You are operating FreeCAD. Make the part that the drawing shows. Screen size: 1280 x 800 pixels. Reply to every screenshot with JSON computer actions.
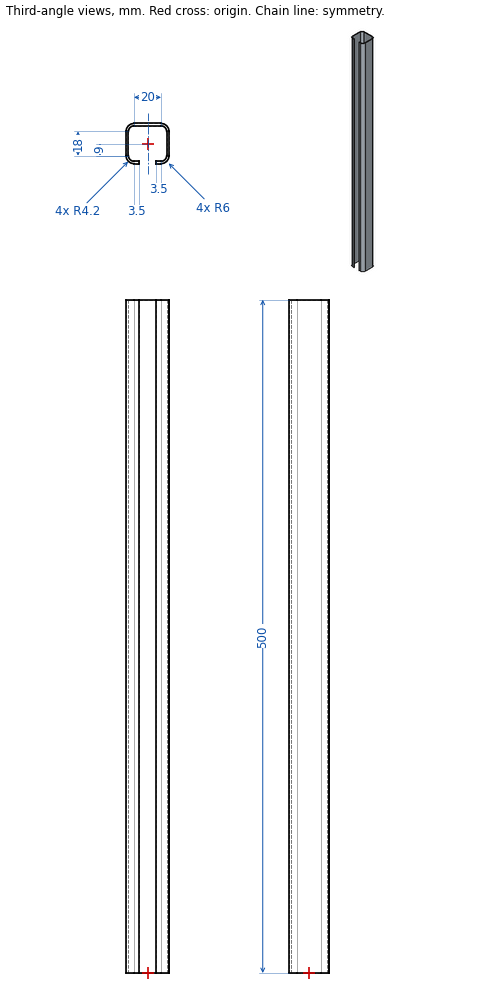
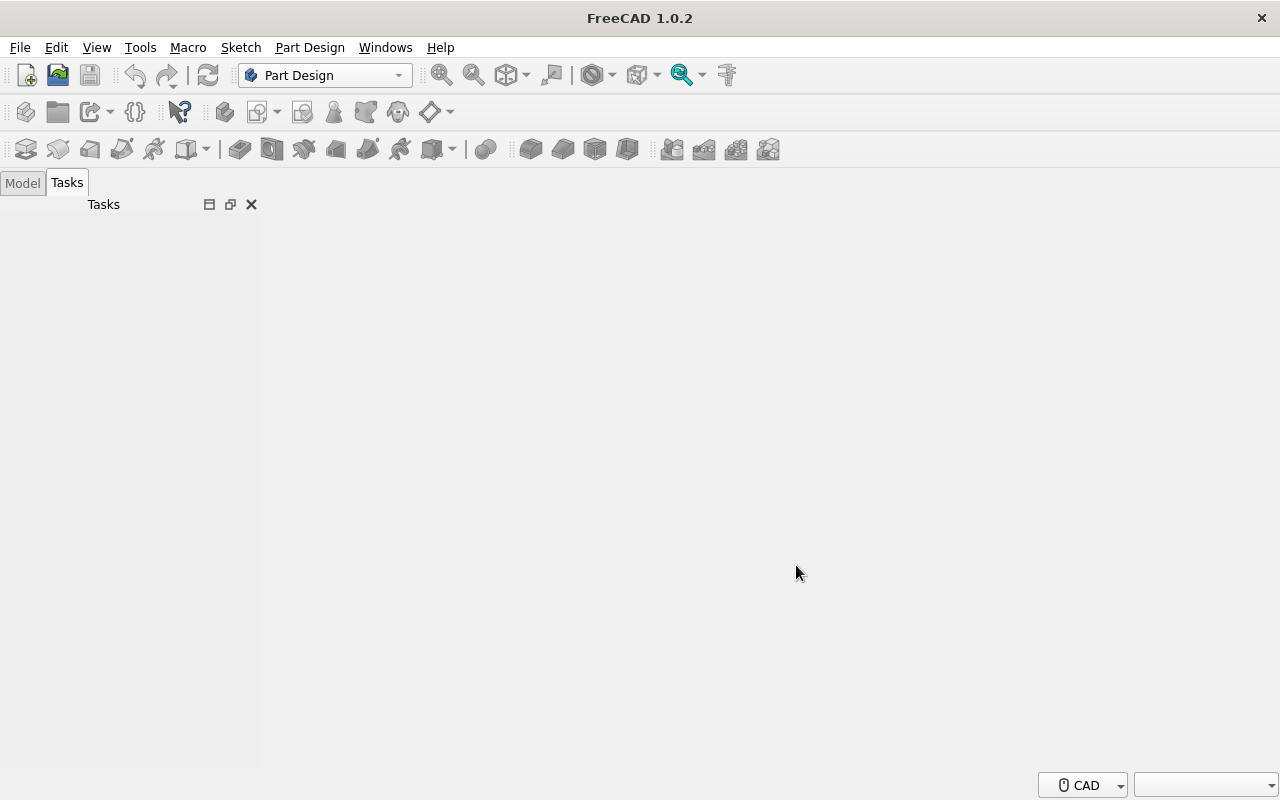
{"action": "left_click", "coordinate": [26, 76]}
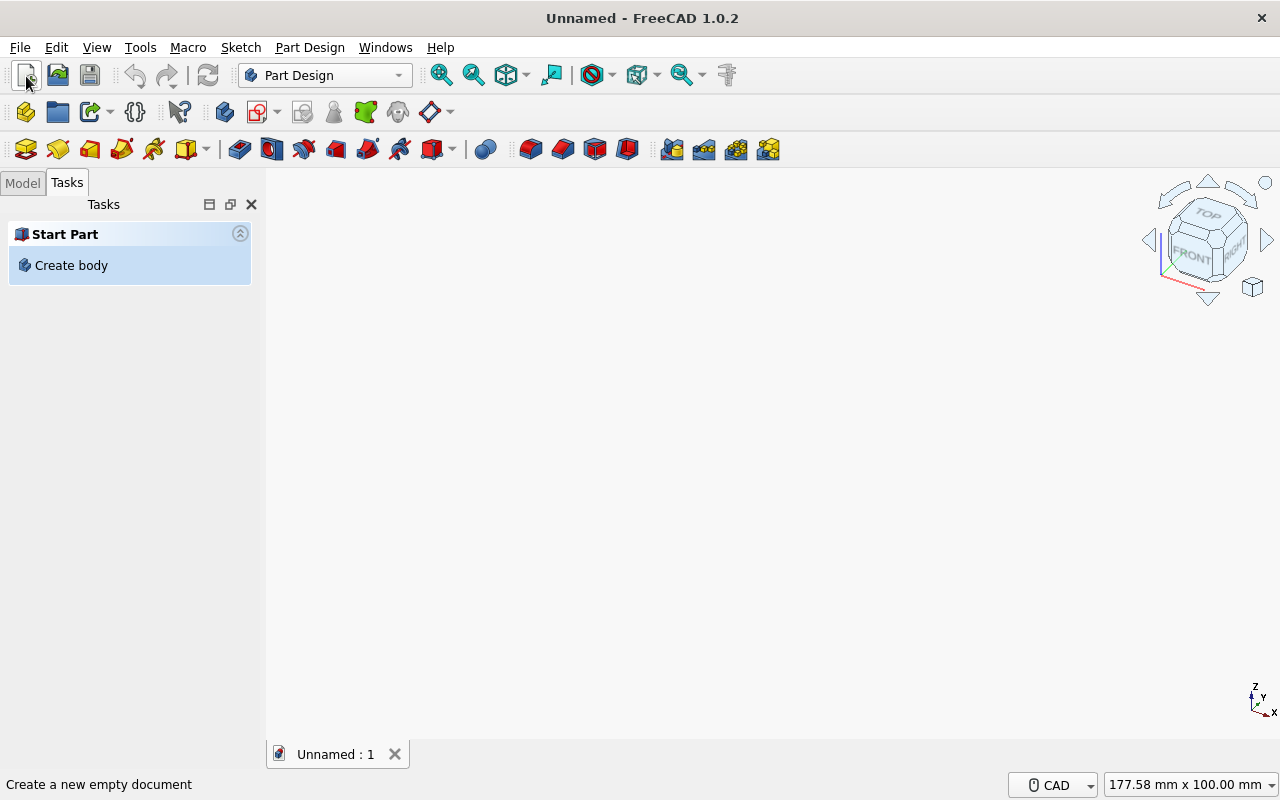
{"action": "left_click", "coordinate": [258, 112]}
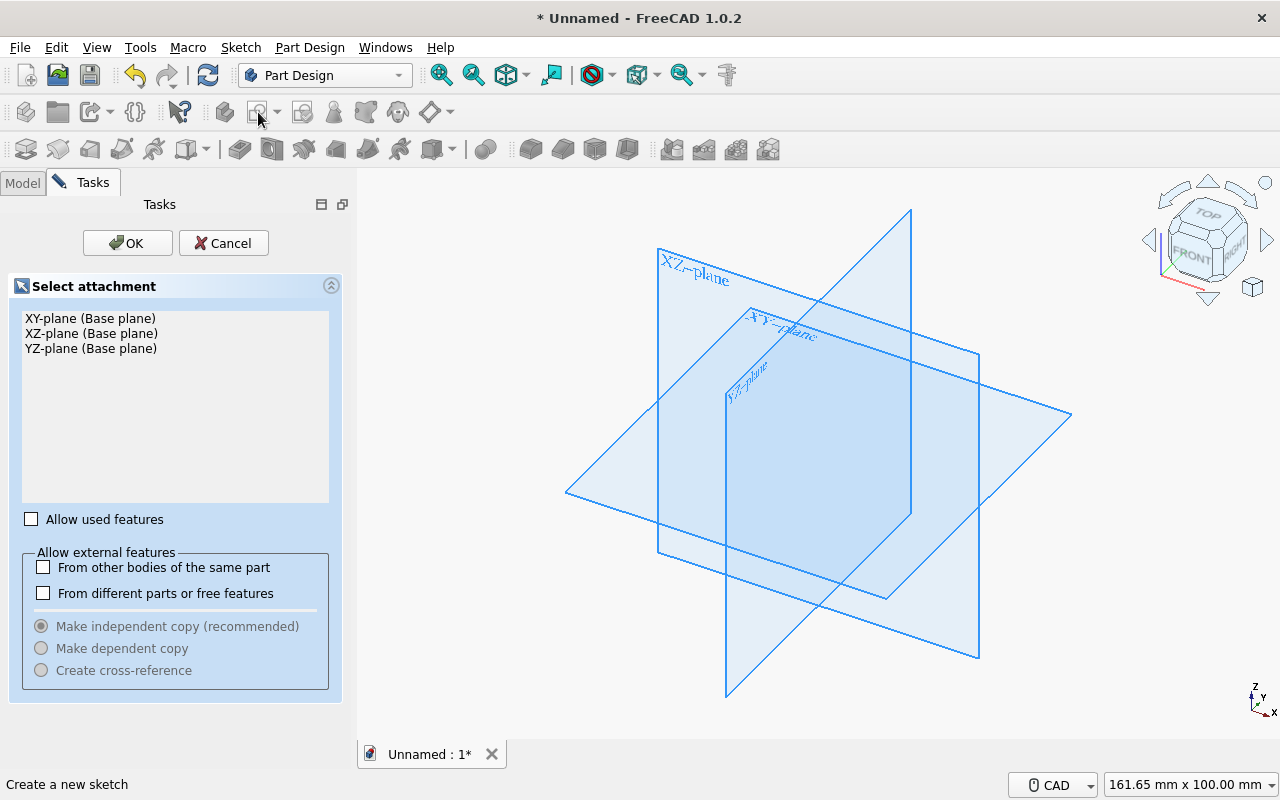
{"action": "left_click", "coordinate": [82, 318]}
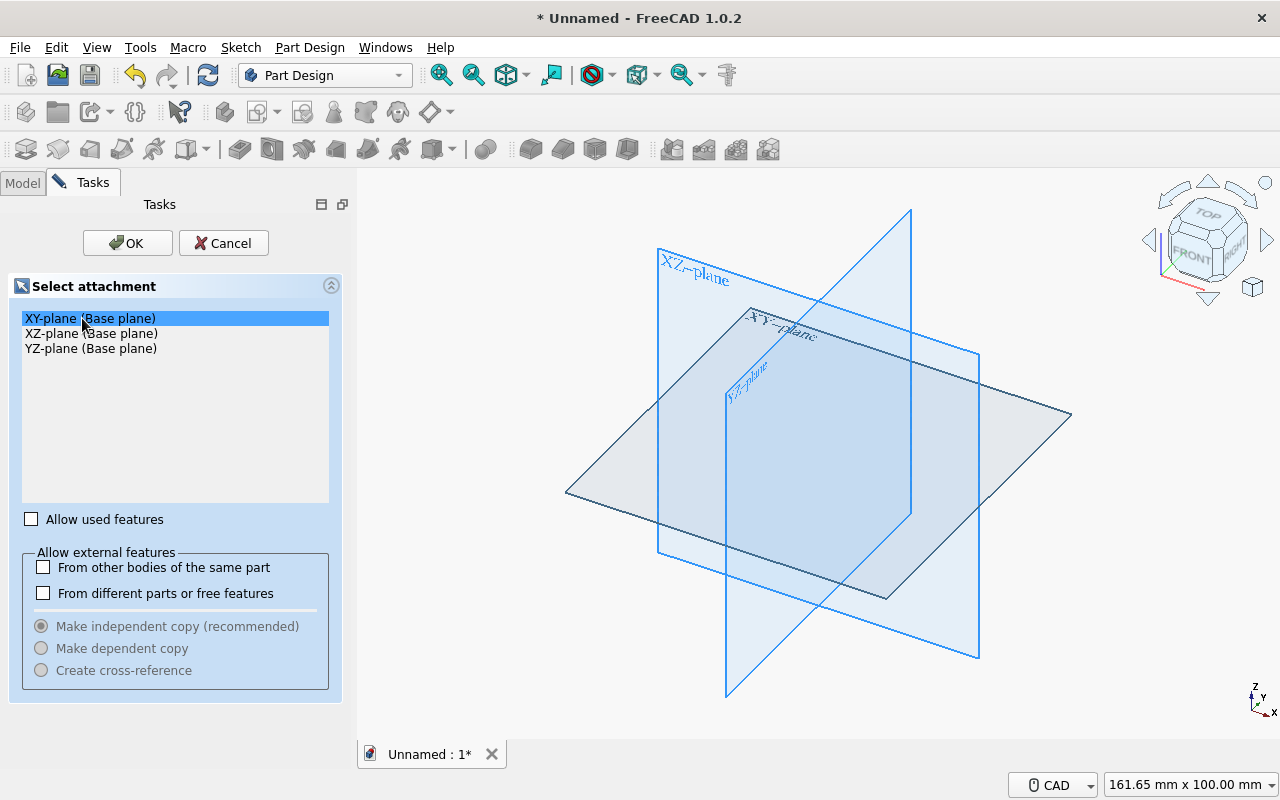
{"action": "left_click", "coordinate": [128, 243]}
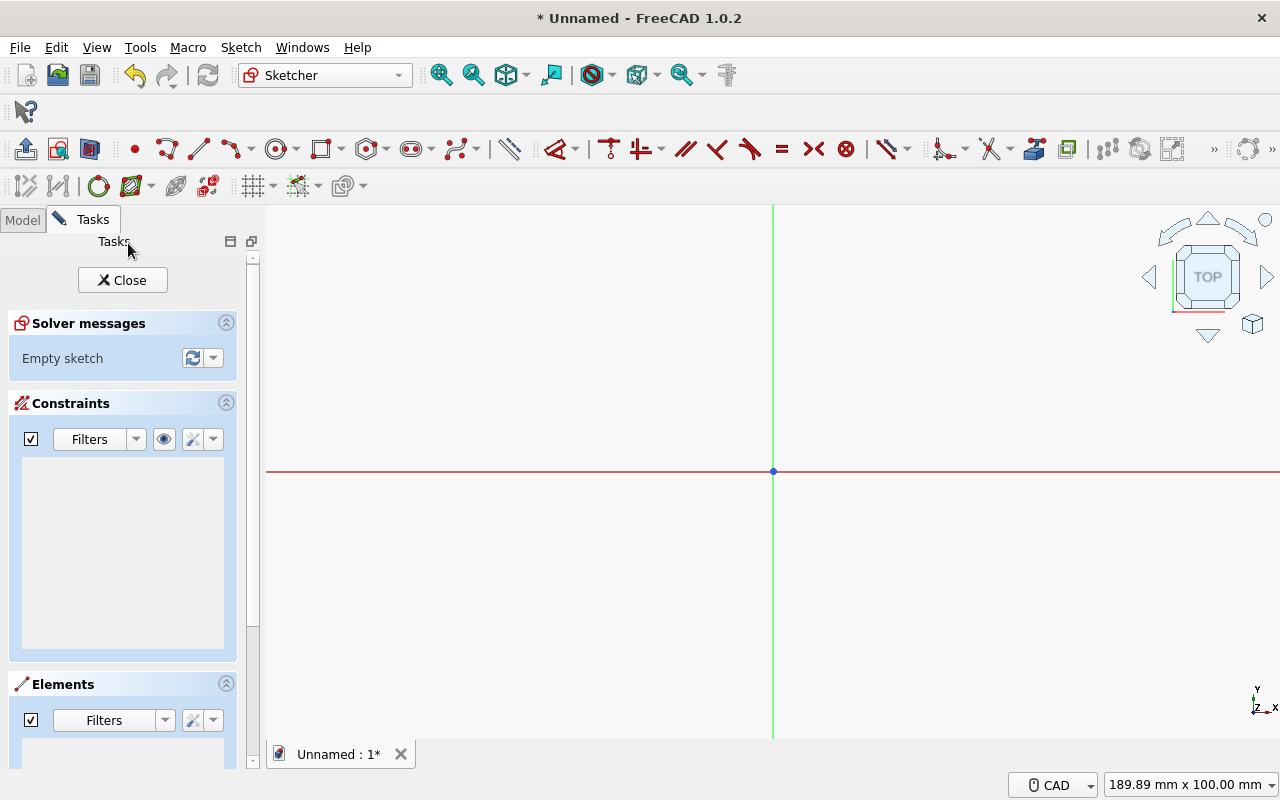
{"action": "scroll", "coordinate": [829, 472], "scroll_direction": "up", "scroll_amount": 4}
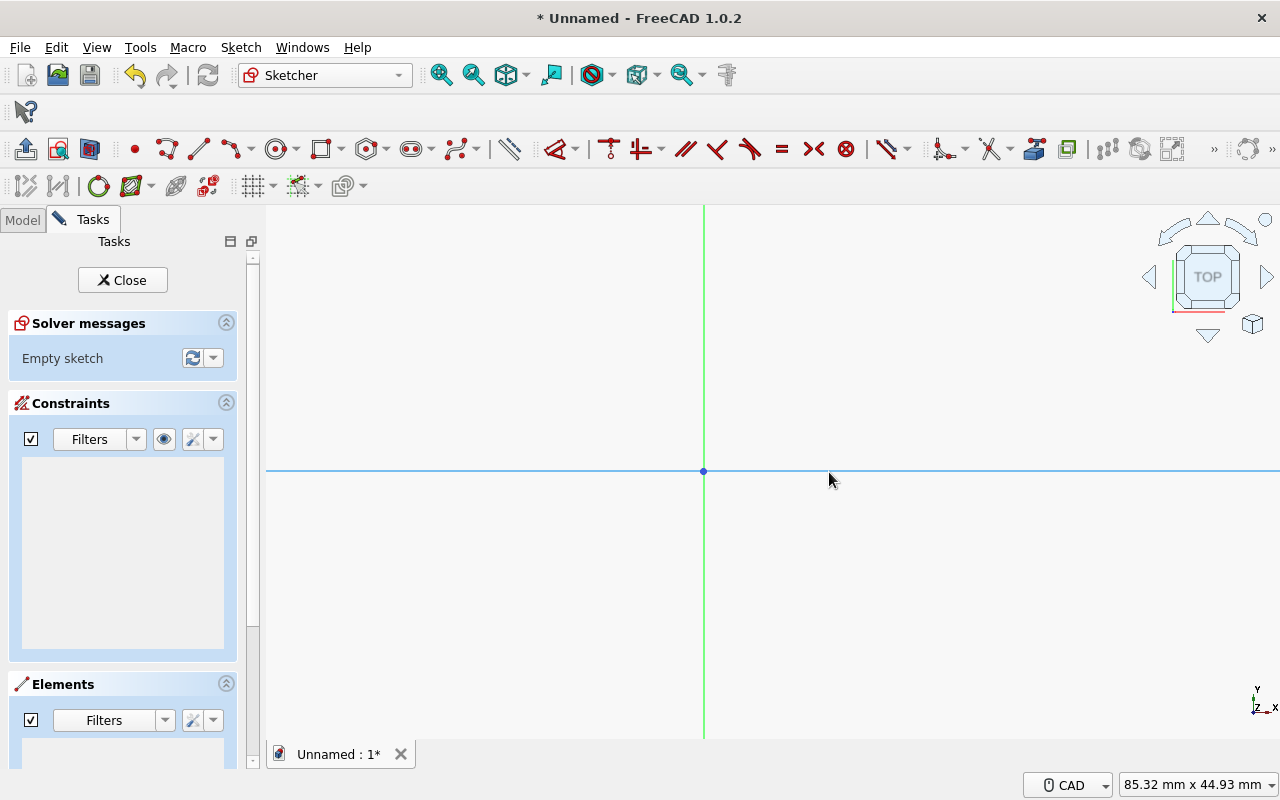
{"action": "left_click", "coordinate": [200, 150]}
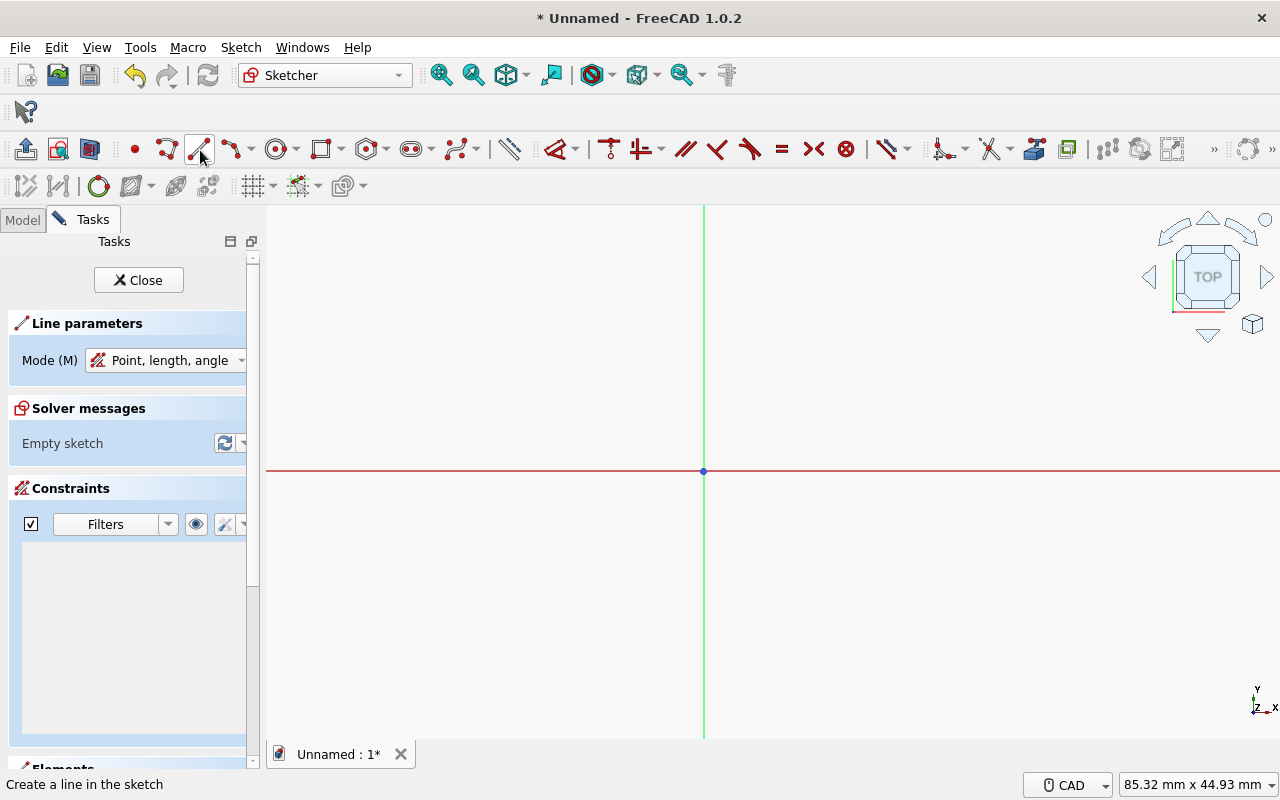
{"action": "left_click", "coordinate": [535, 578]}
{"action": "left_click", "coordinate": [535, 364]}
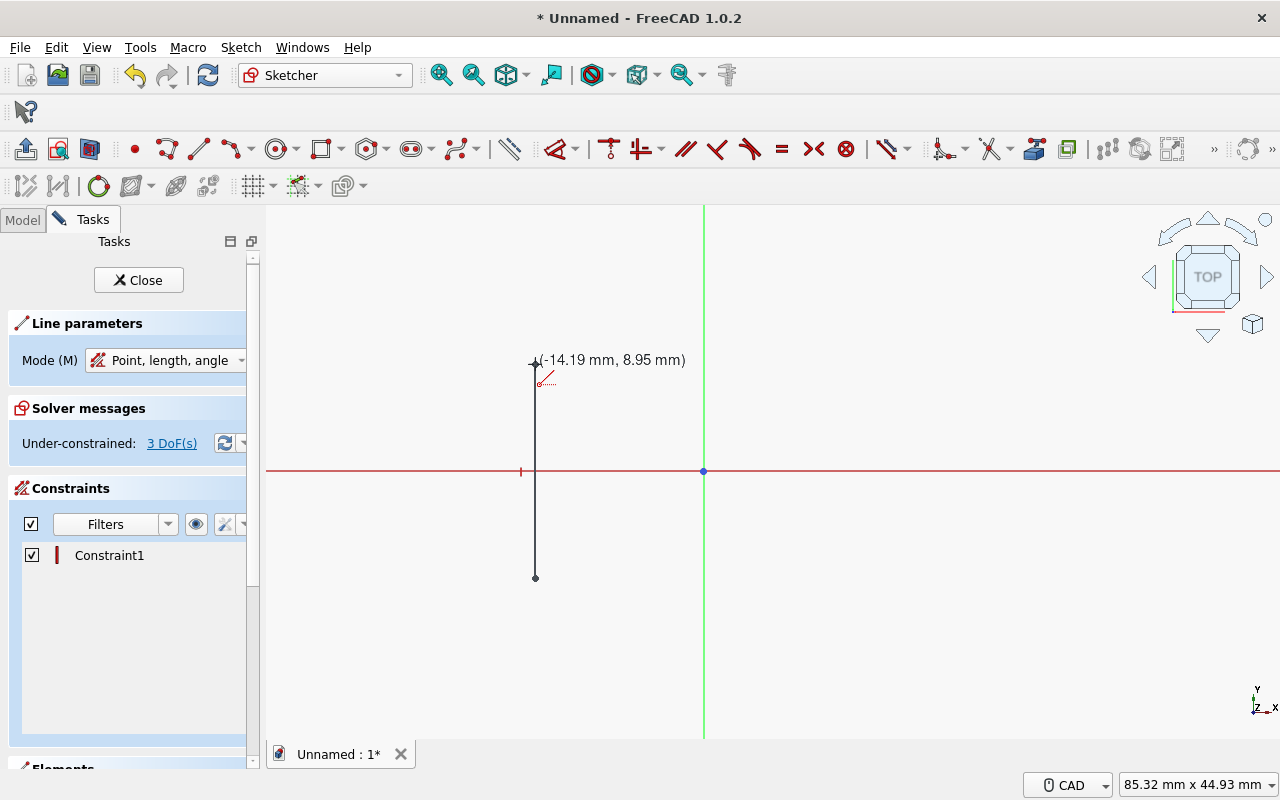
{"action": "left_click", "coordinate": [585, 315]}
{"action": "left_click", "coordinate": [823, 315]}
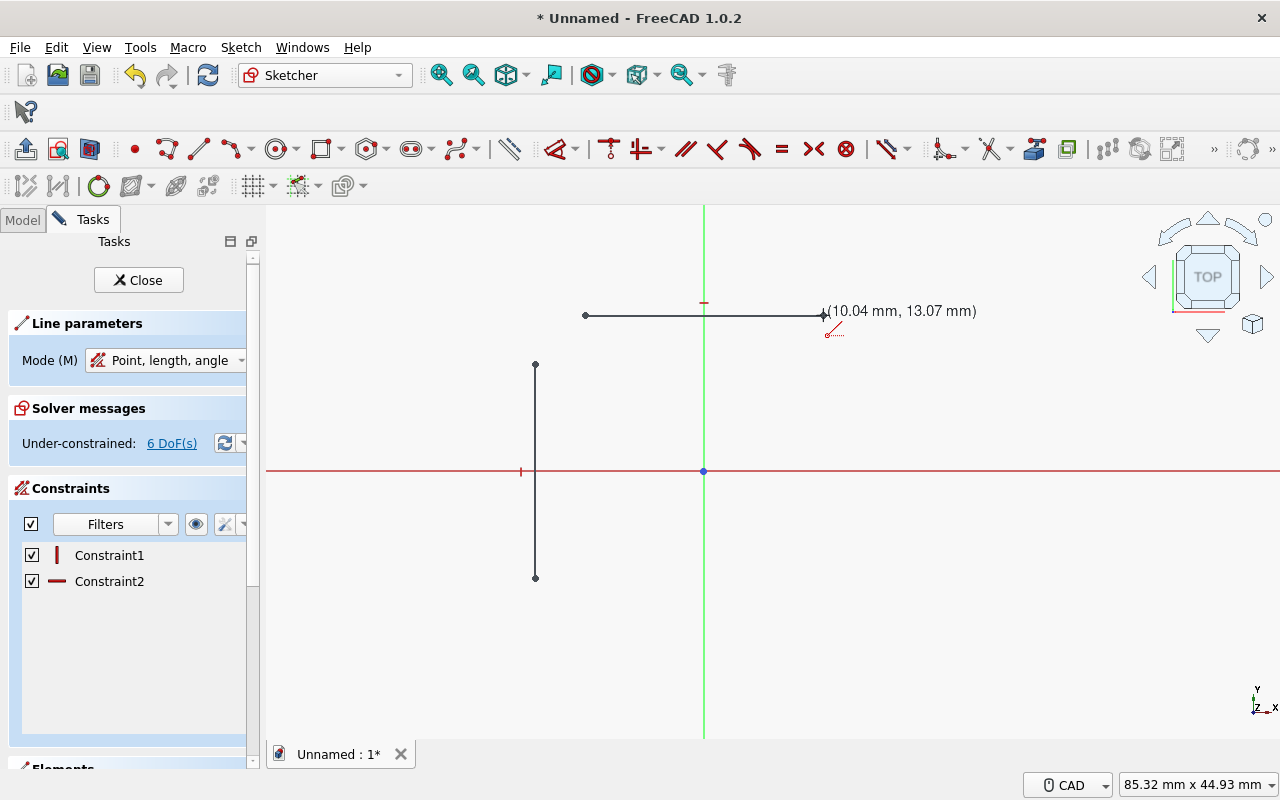
{"action": "left_click", "coordinate": [872, 364]}
{"action": "left_click", "coordinate": [872, 578]}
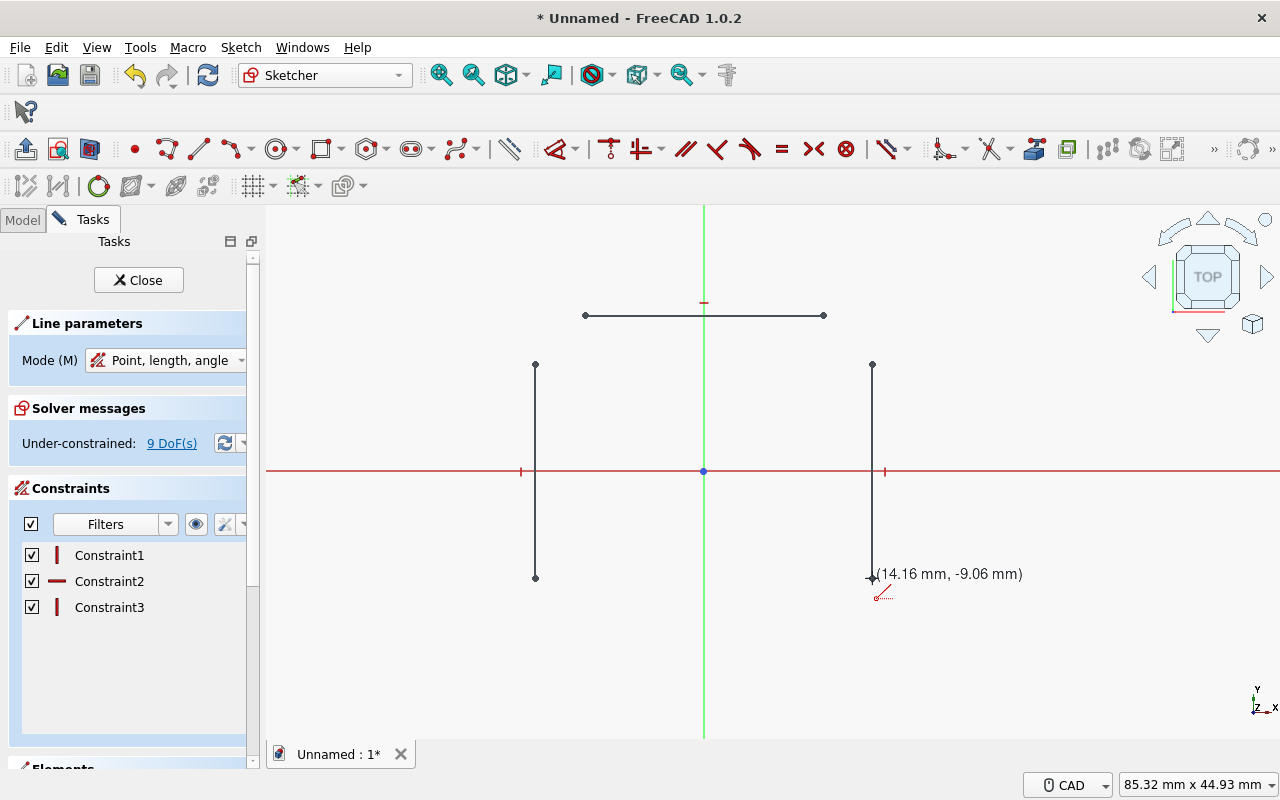
{"action": "left_click", "coordinate": [168, 150]}